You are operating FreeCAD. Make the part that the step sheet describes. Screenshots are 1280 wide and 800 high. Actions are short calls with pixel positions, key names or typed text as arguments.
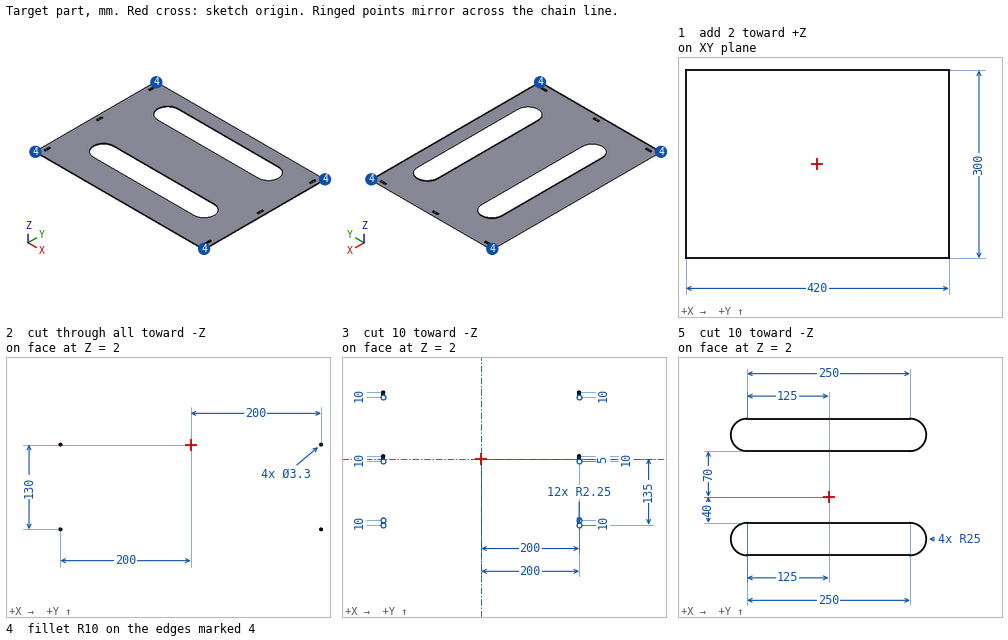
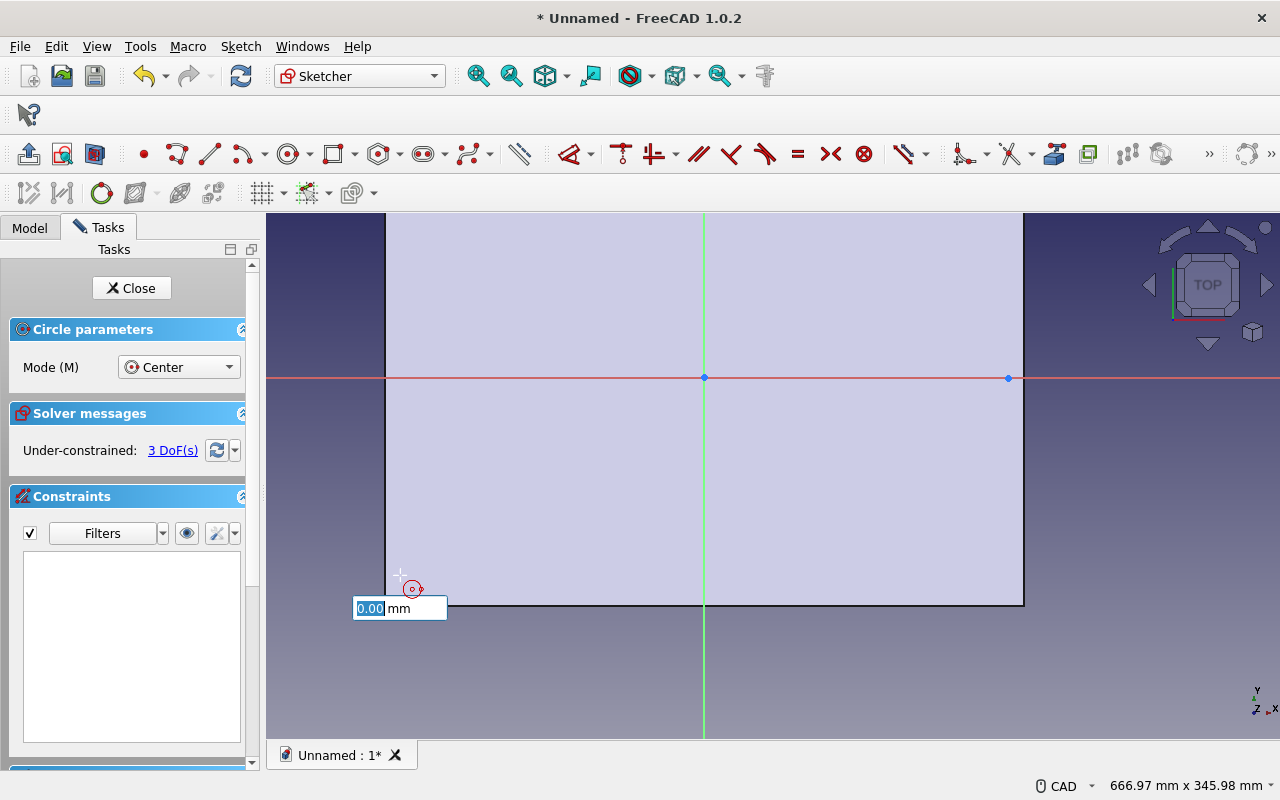
scroll(402, 573, up, 10)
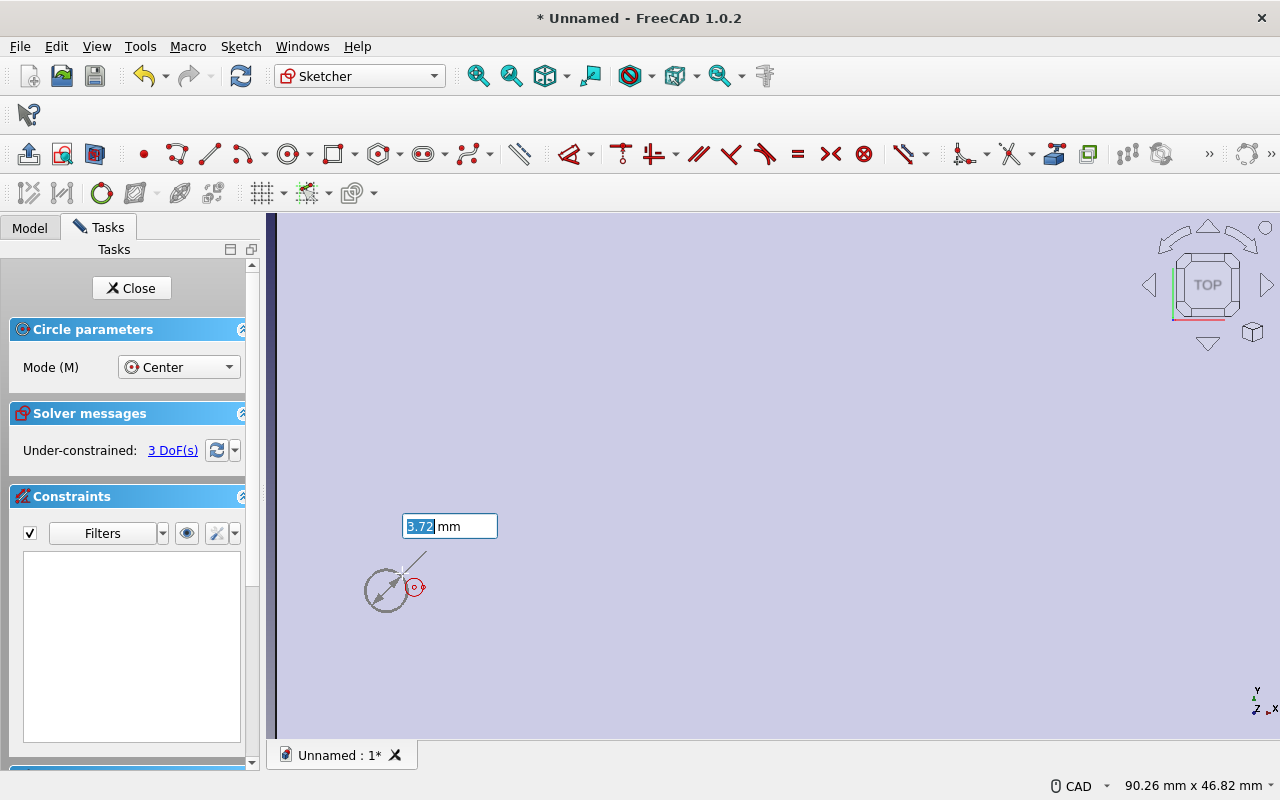
click(401, 572)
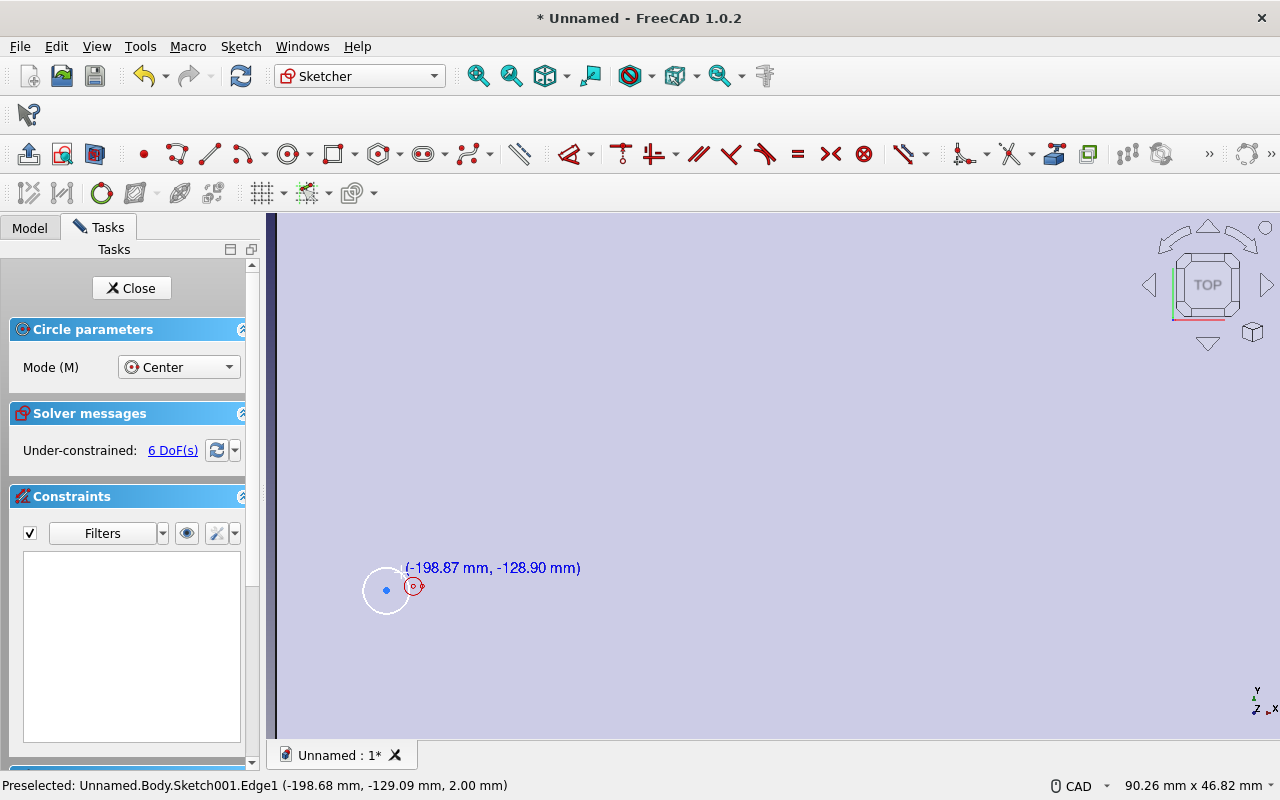
scroll(402, 573, down, 10)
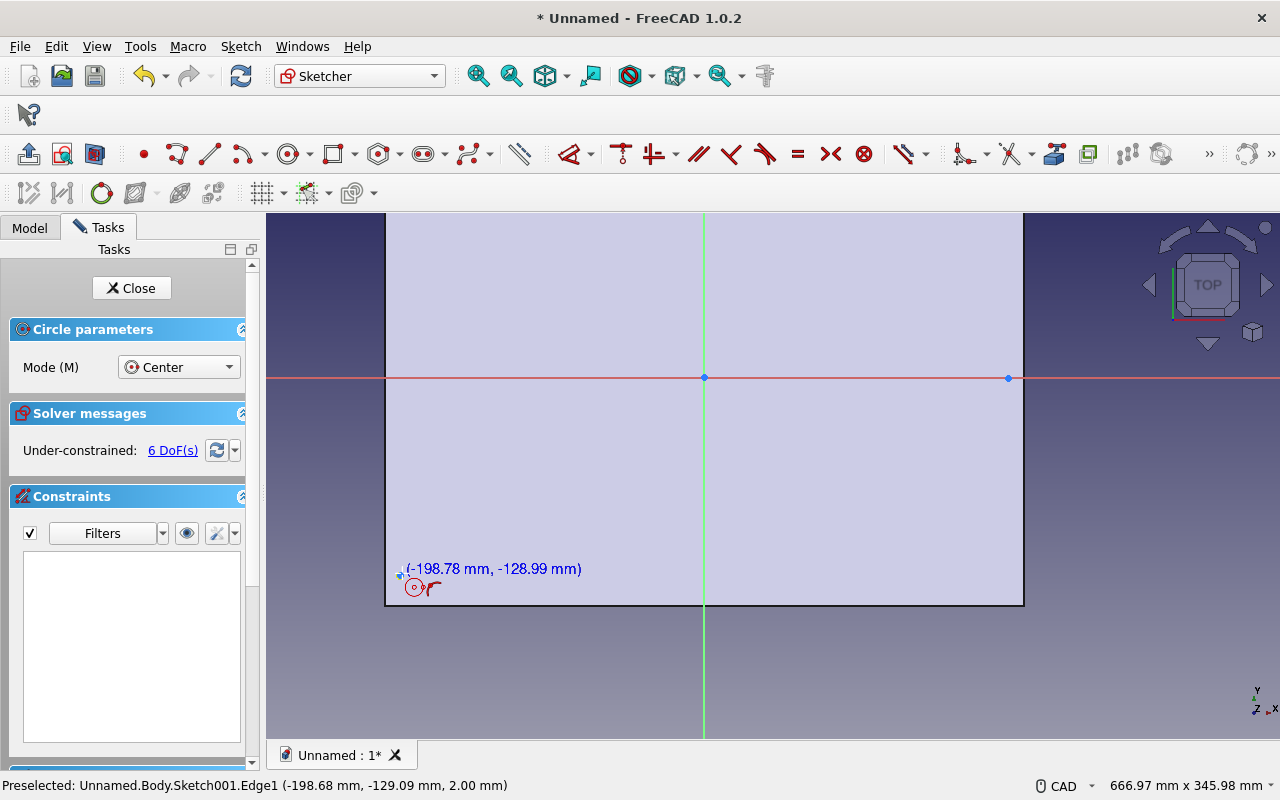
scroll(400, 378, up, 12)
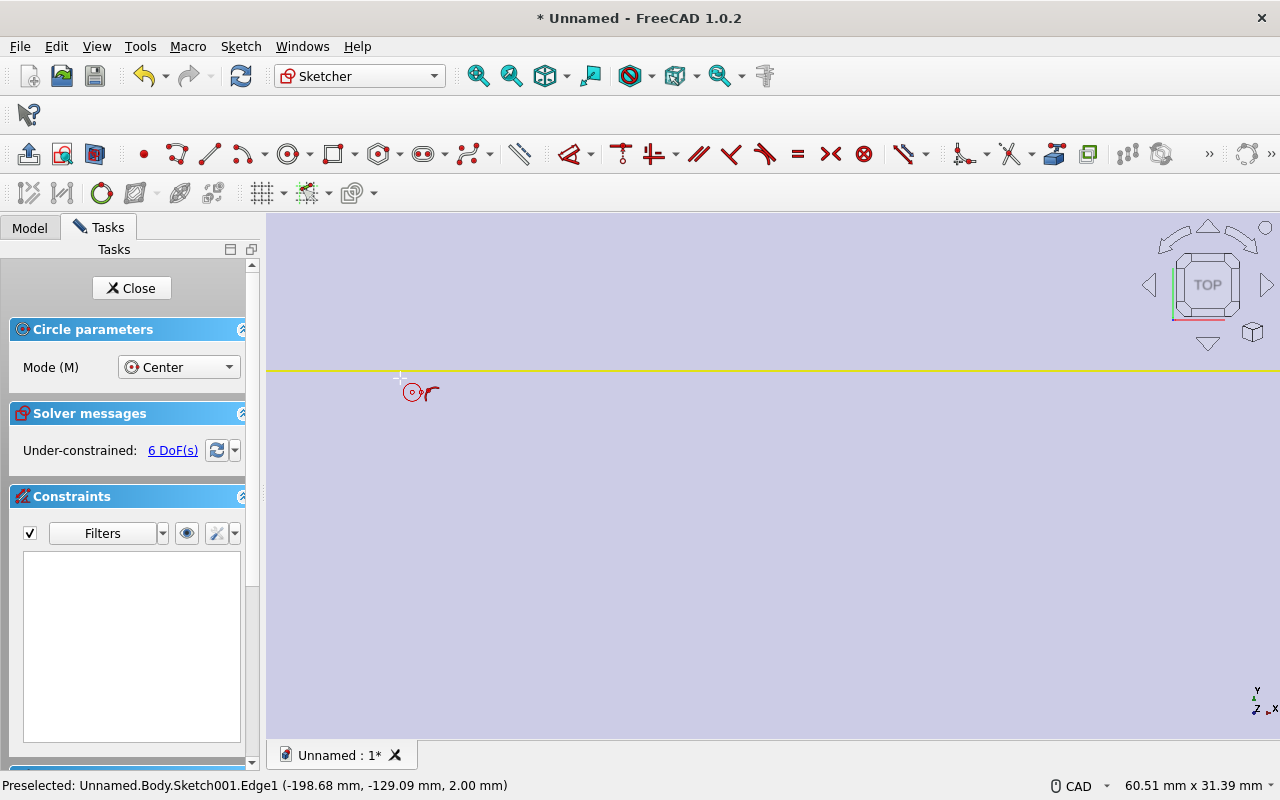
scroll(400, 378, down, 12)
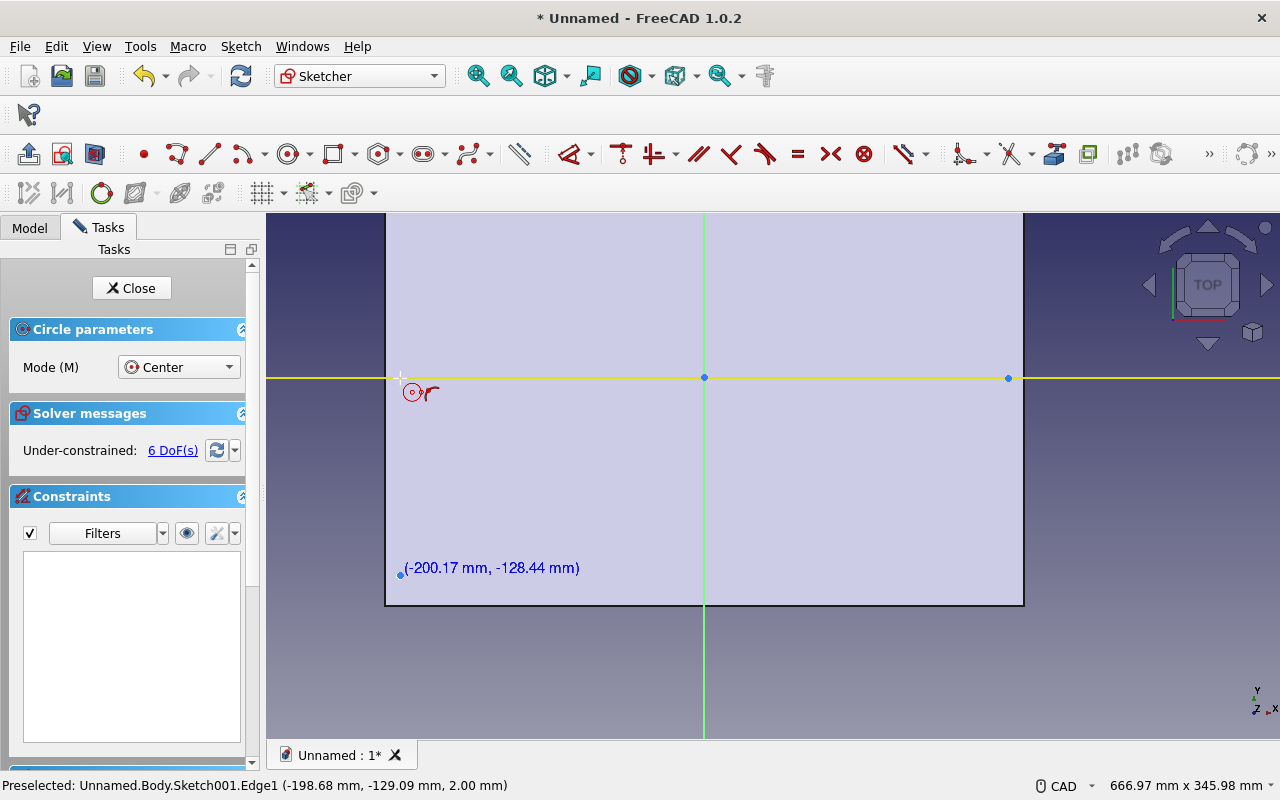
click(400, 378)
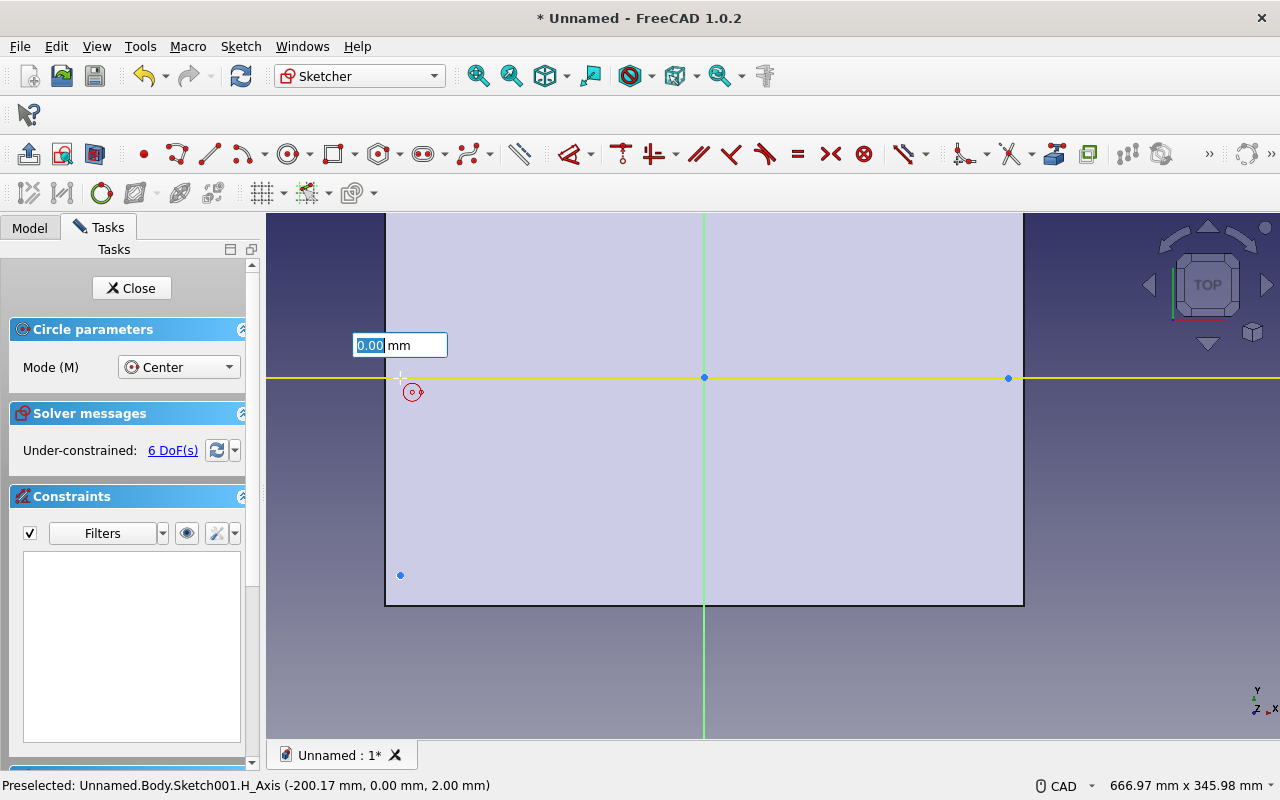
scroll(401, 375, up, 10)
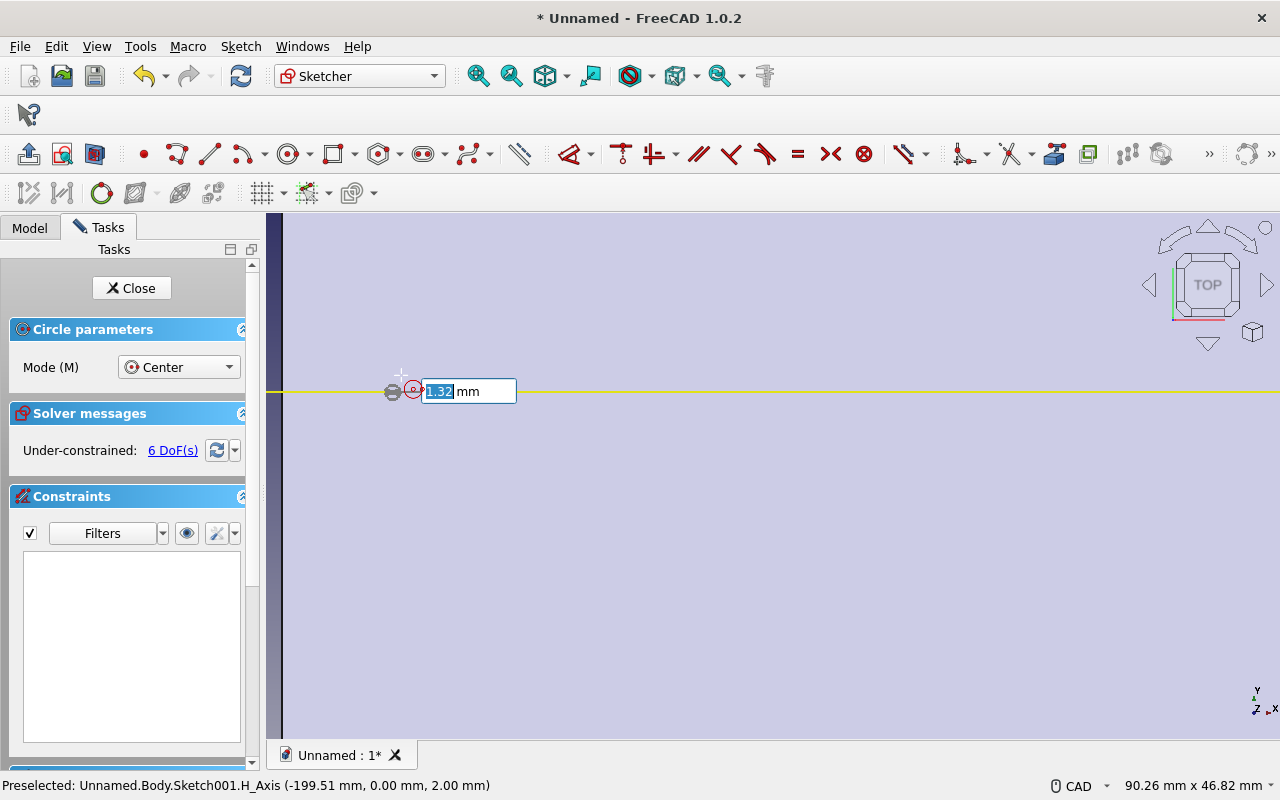
click(401, 375)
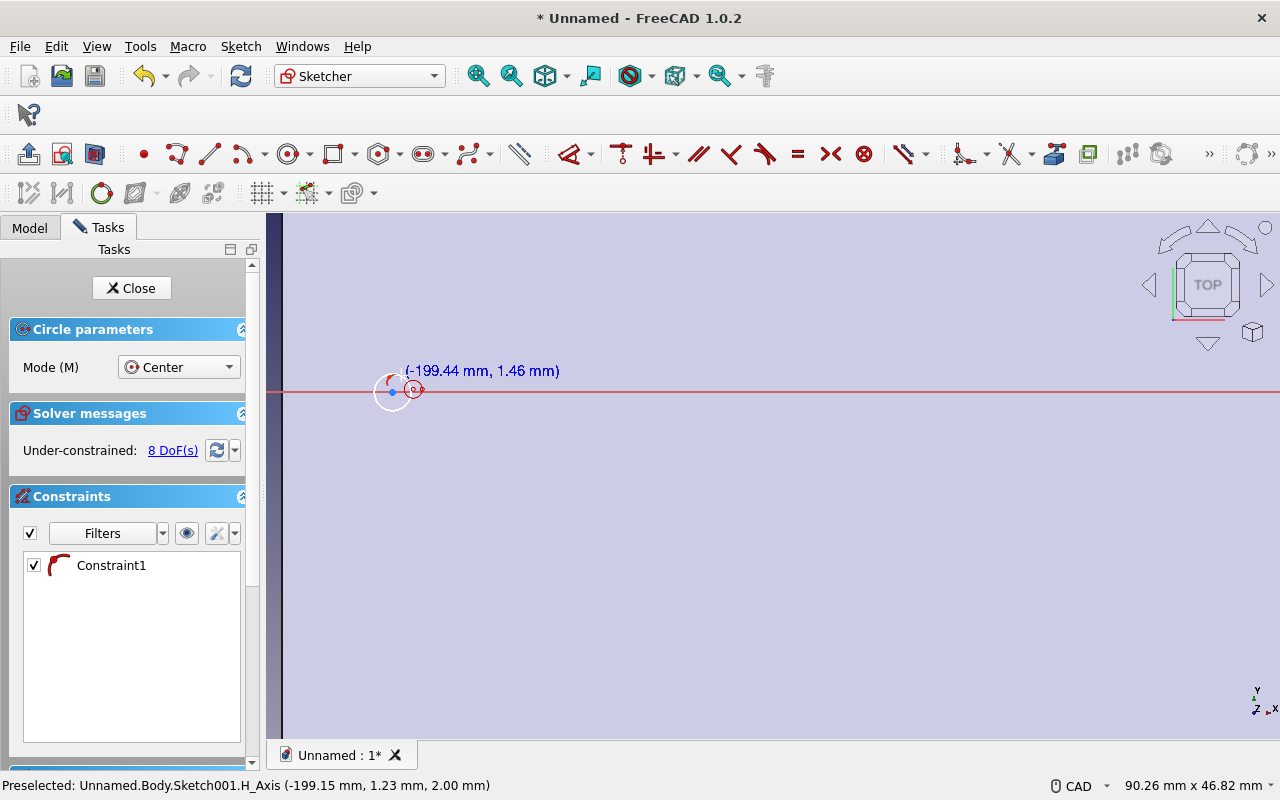
scroll(401, 375, down, 10)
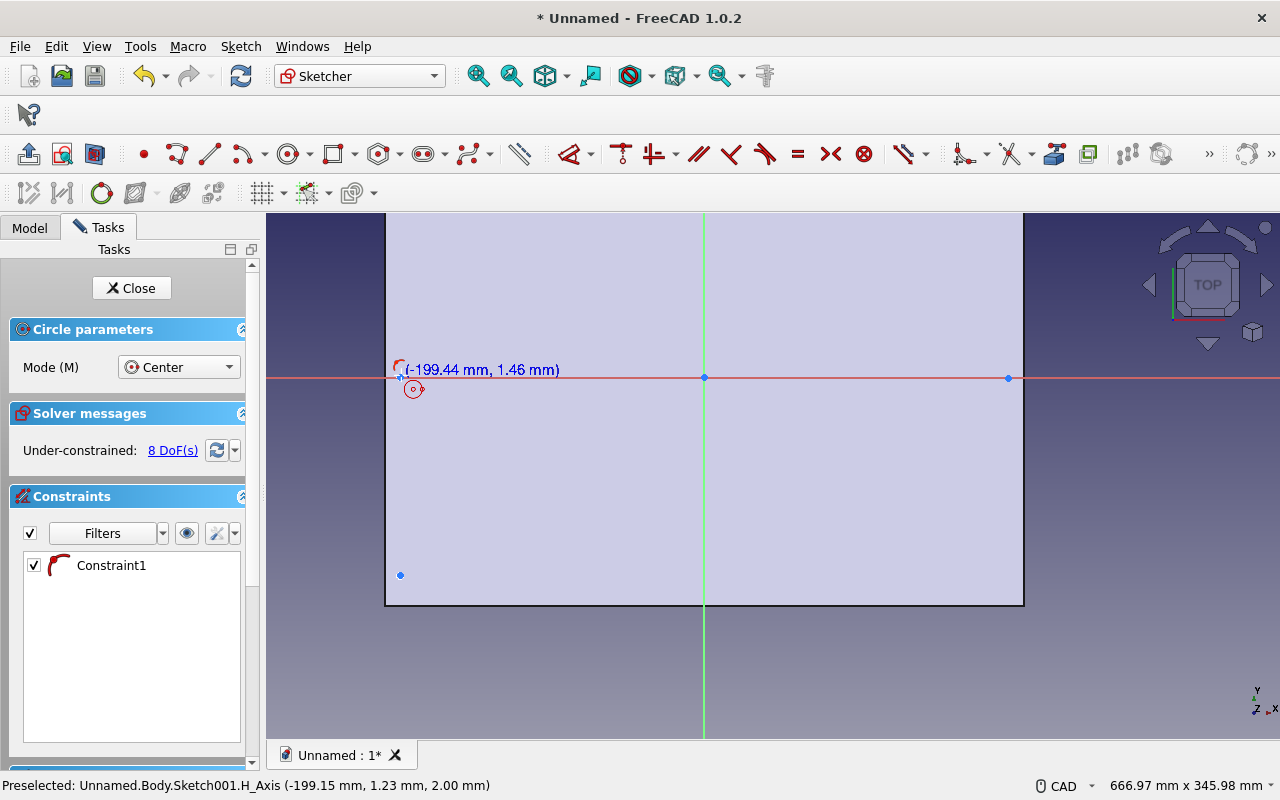
scroll(1008, 575, up, 12)